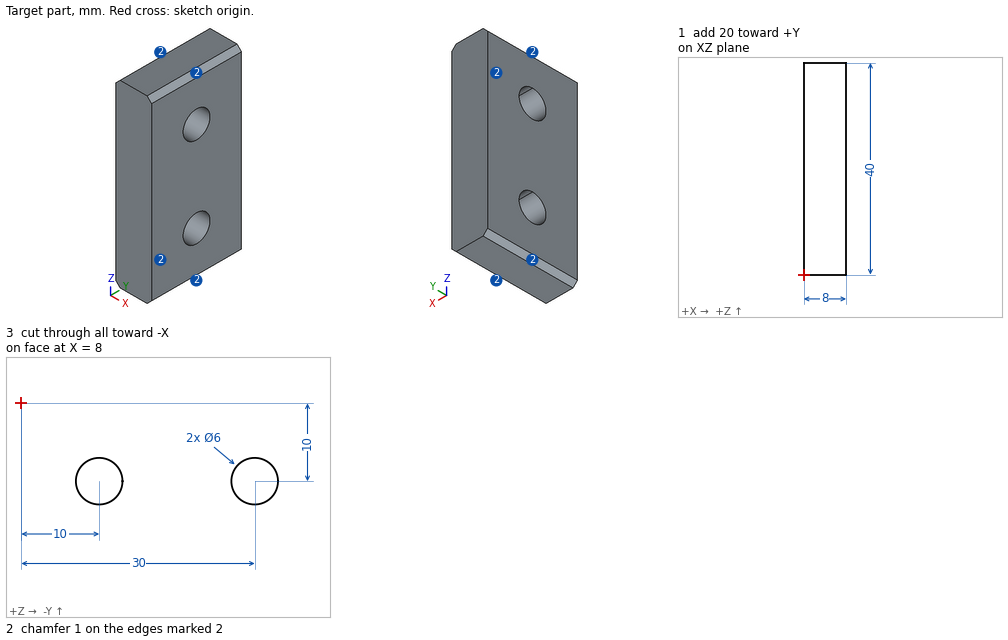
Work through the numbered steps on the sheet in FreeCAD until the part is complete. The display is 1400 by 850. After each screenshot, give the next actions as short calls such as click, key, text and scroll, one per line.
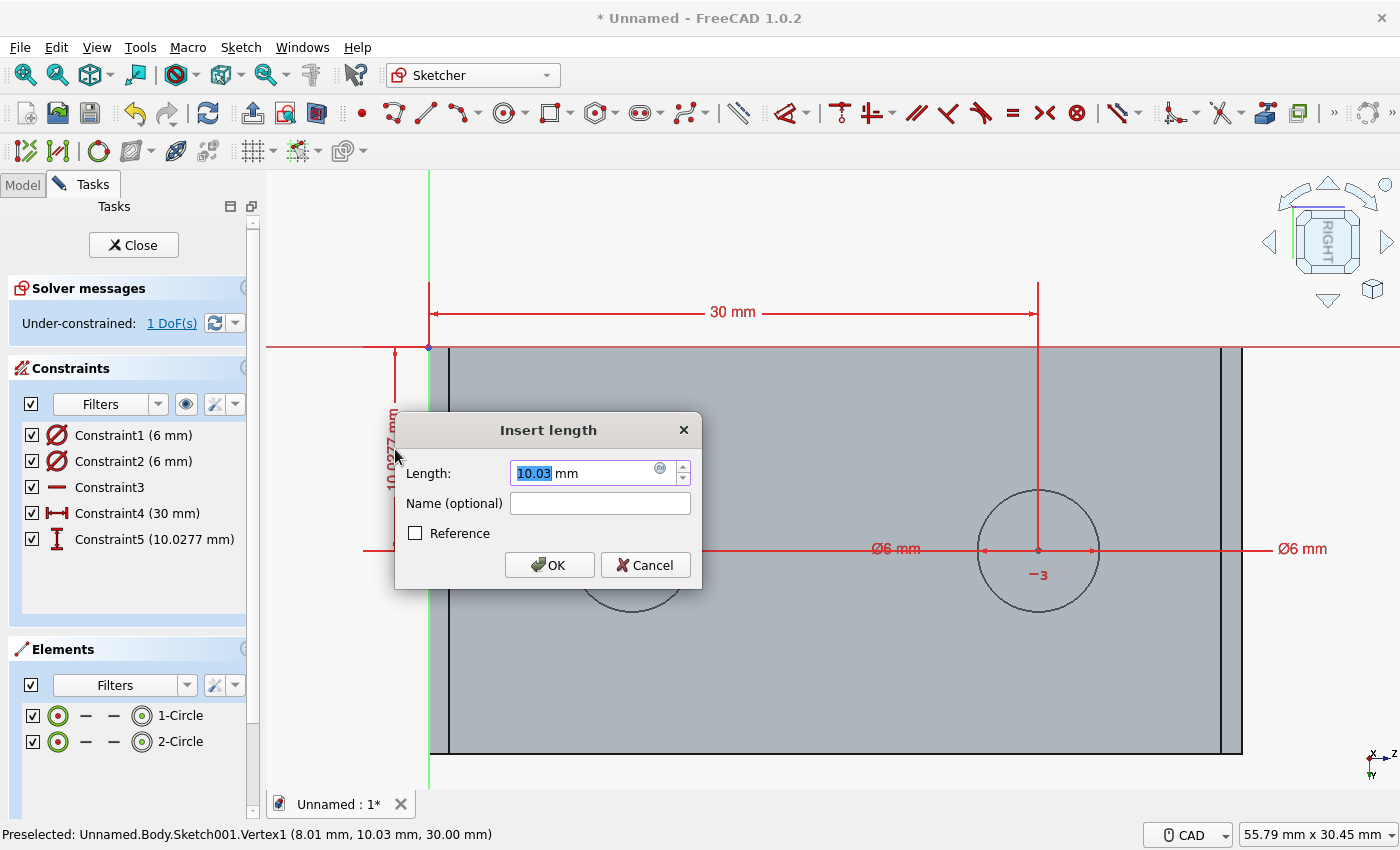
text(10)
key(Return)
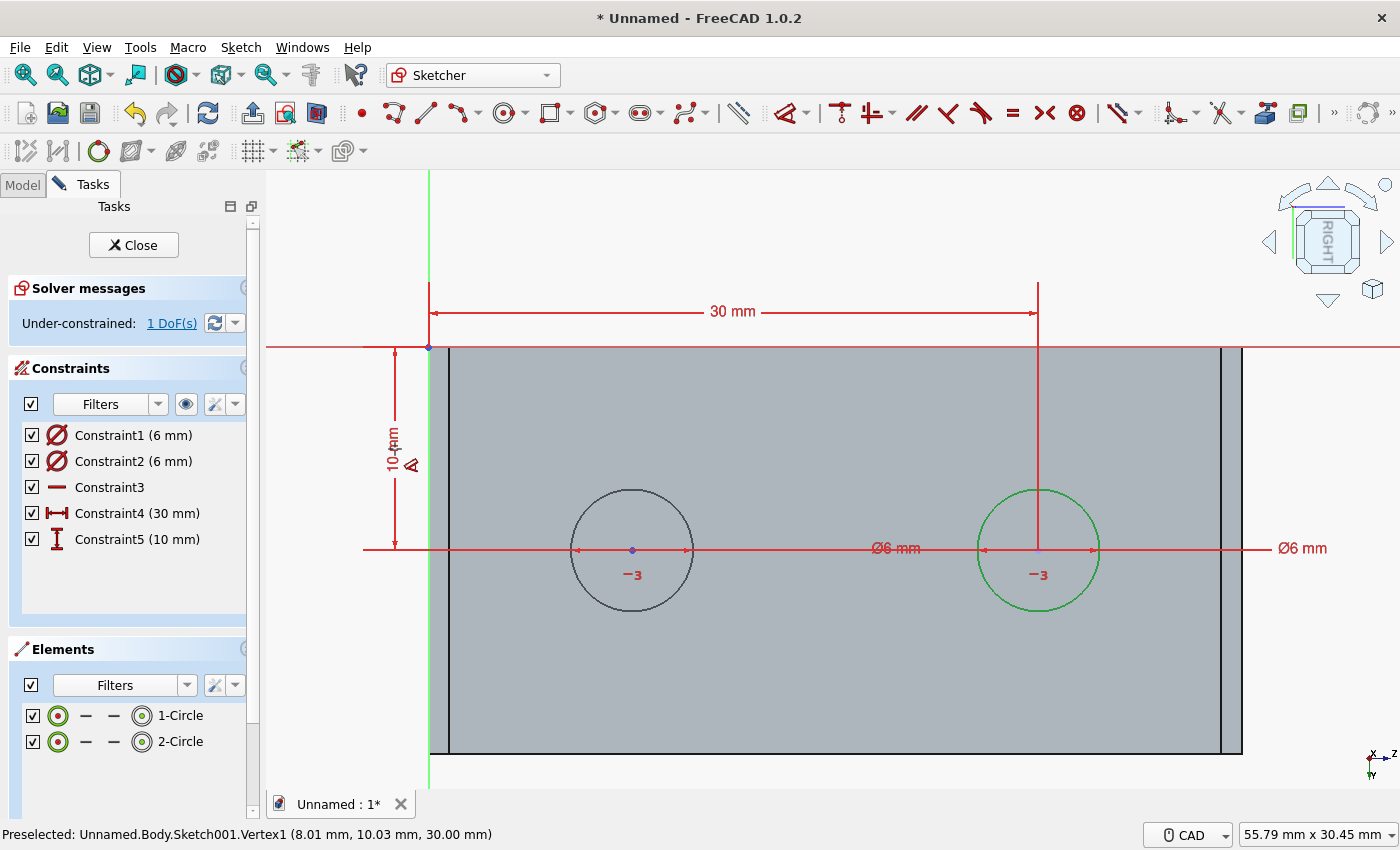
click(632, 550)
click(530, 313)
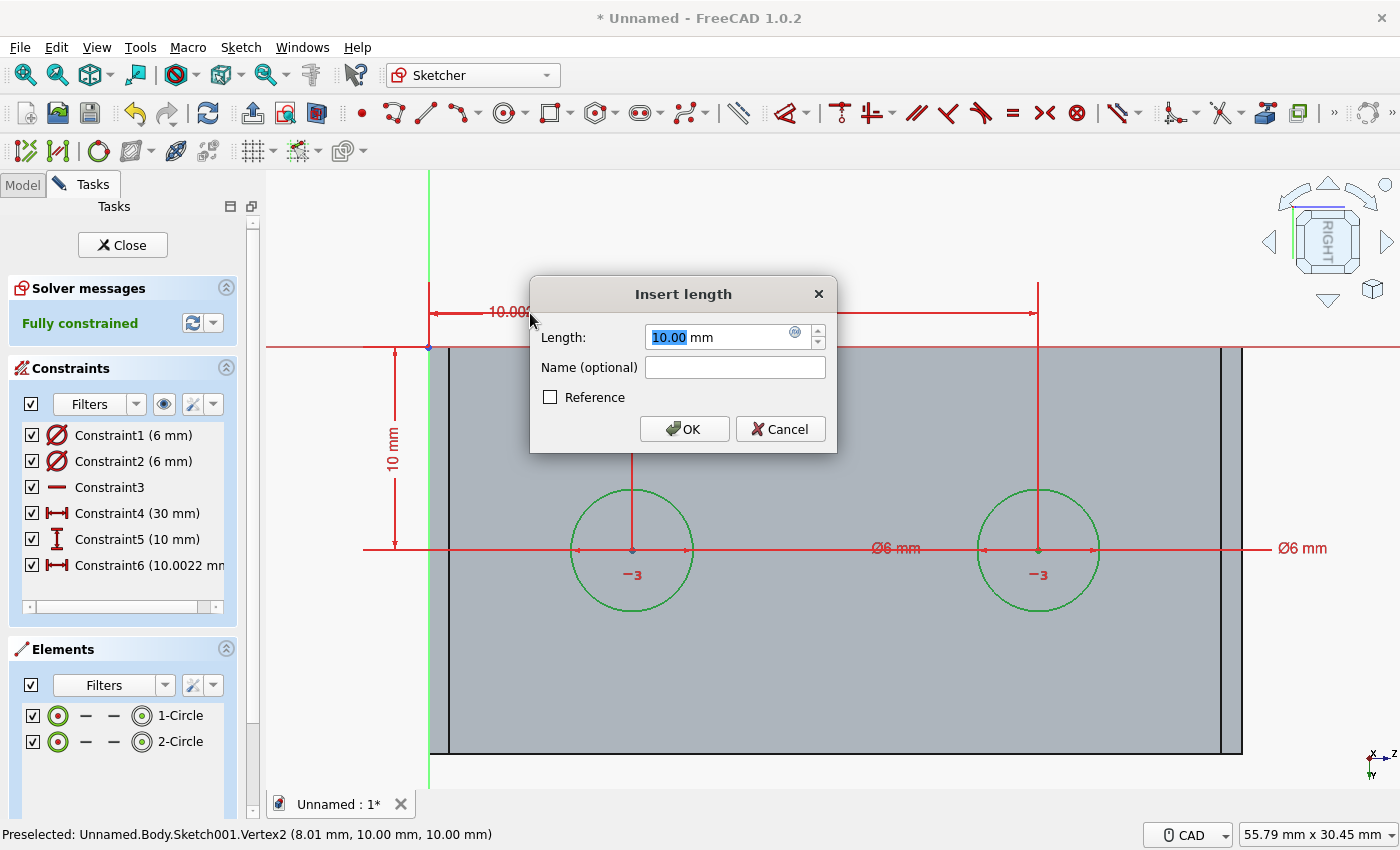
text(10)
key(Return)
key(Escape)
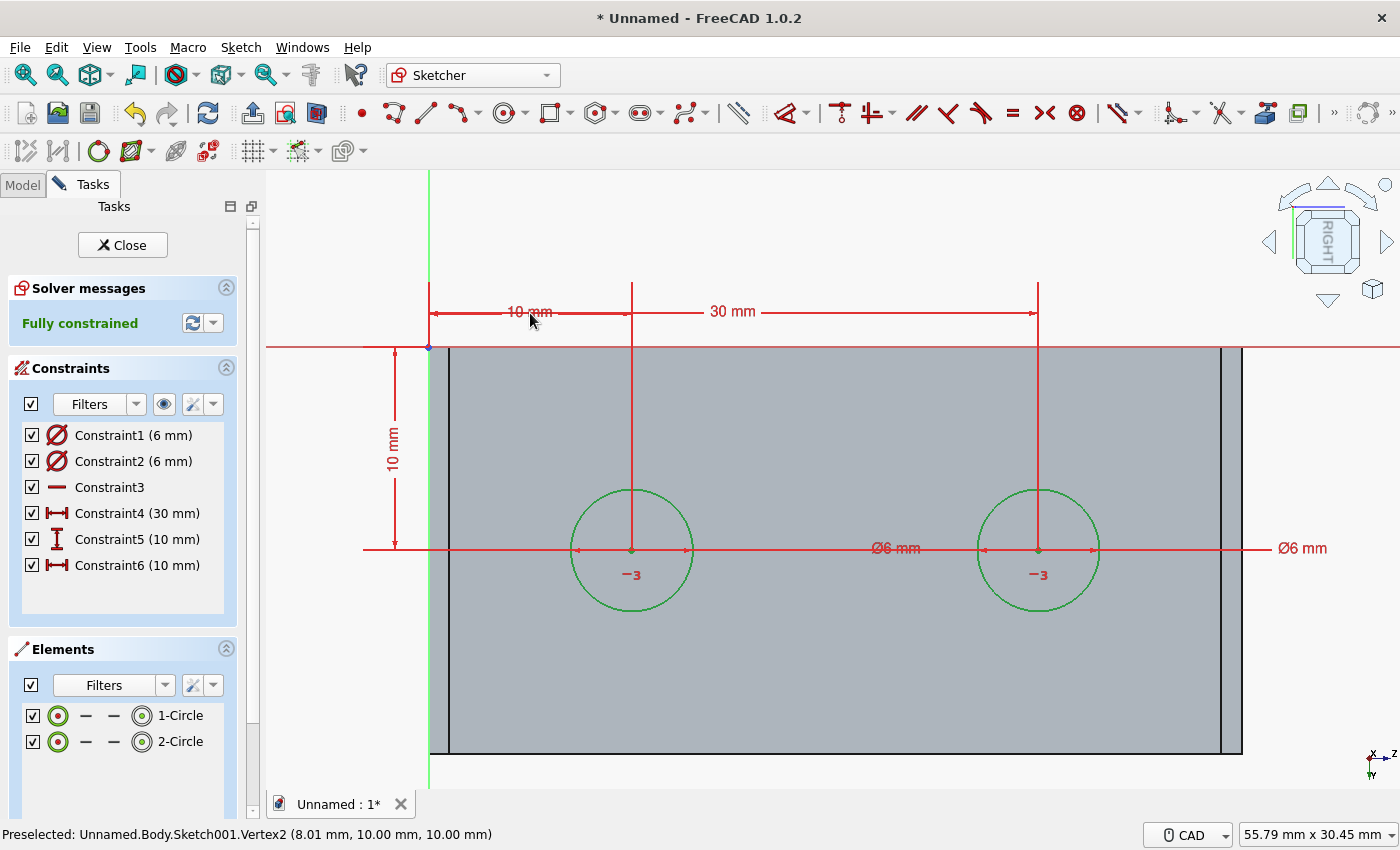
click(123, 245)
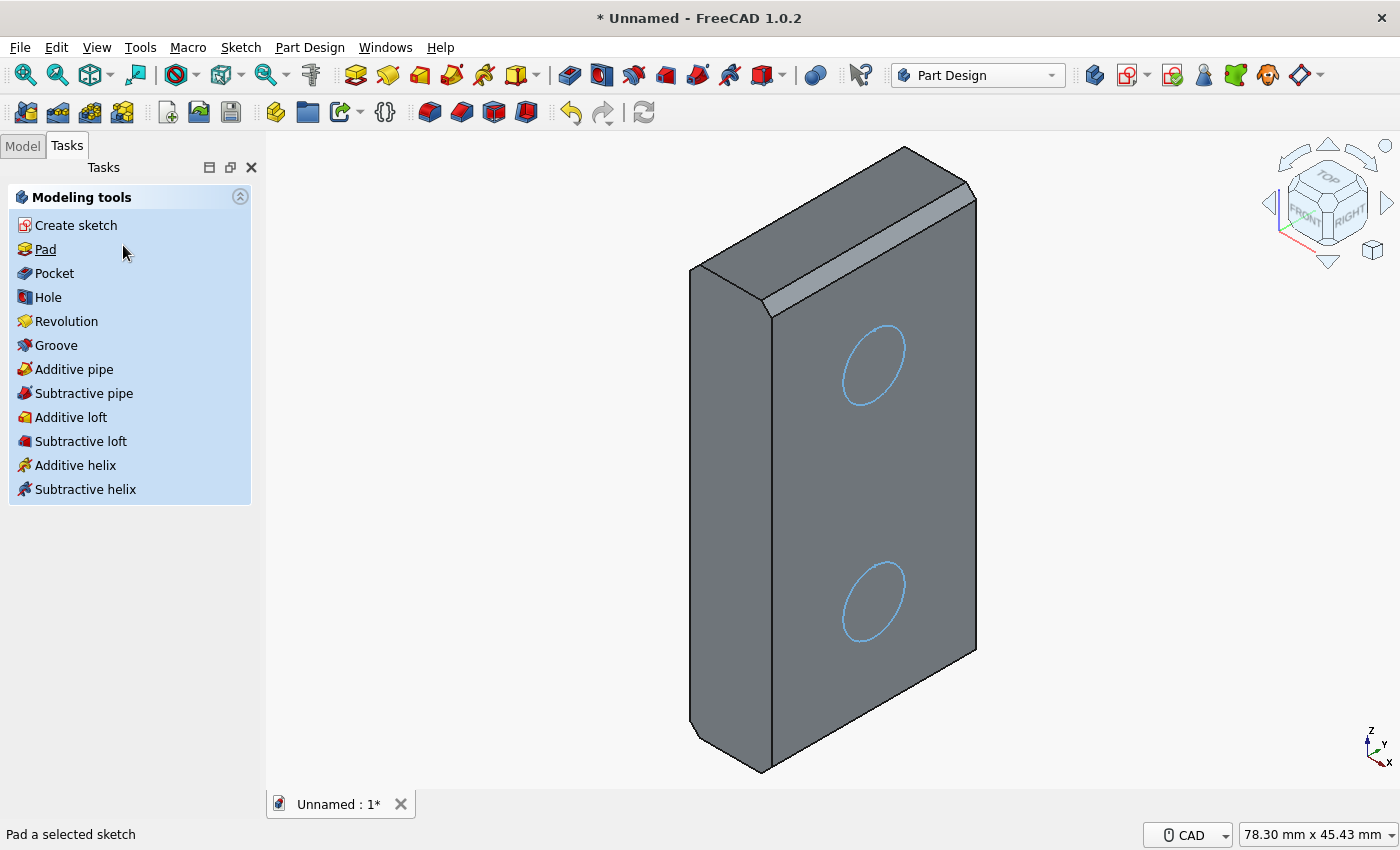
click(570, 76)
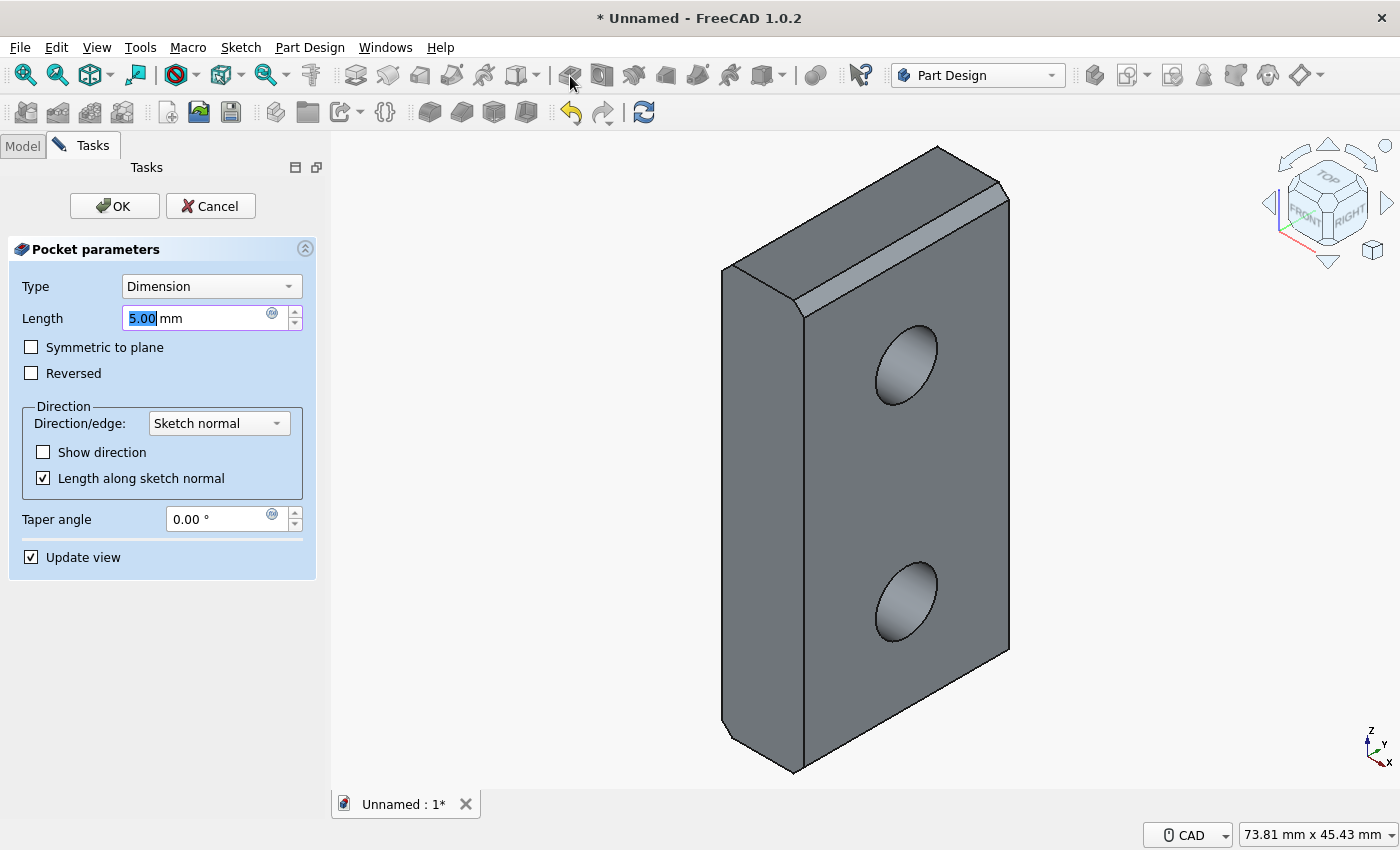
click(212, 286)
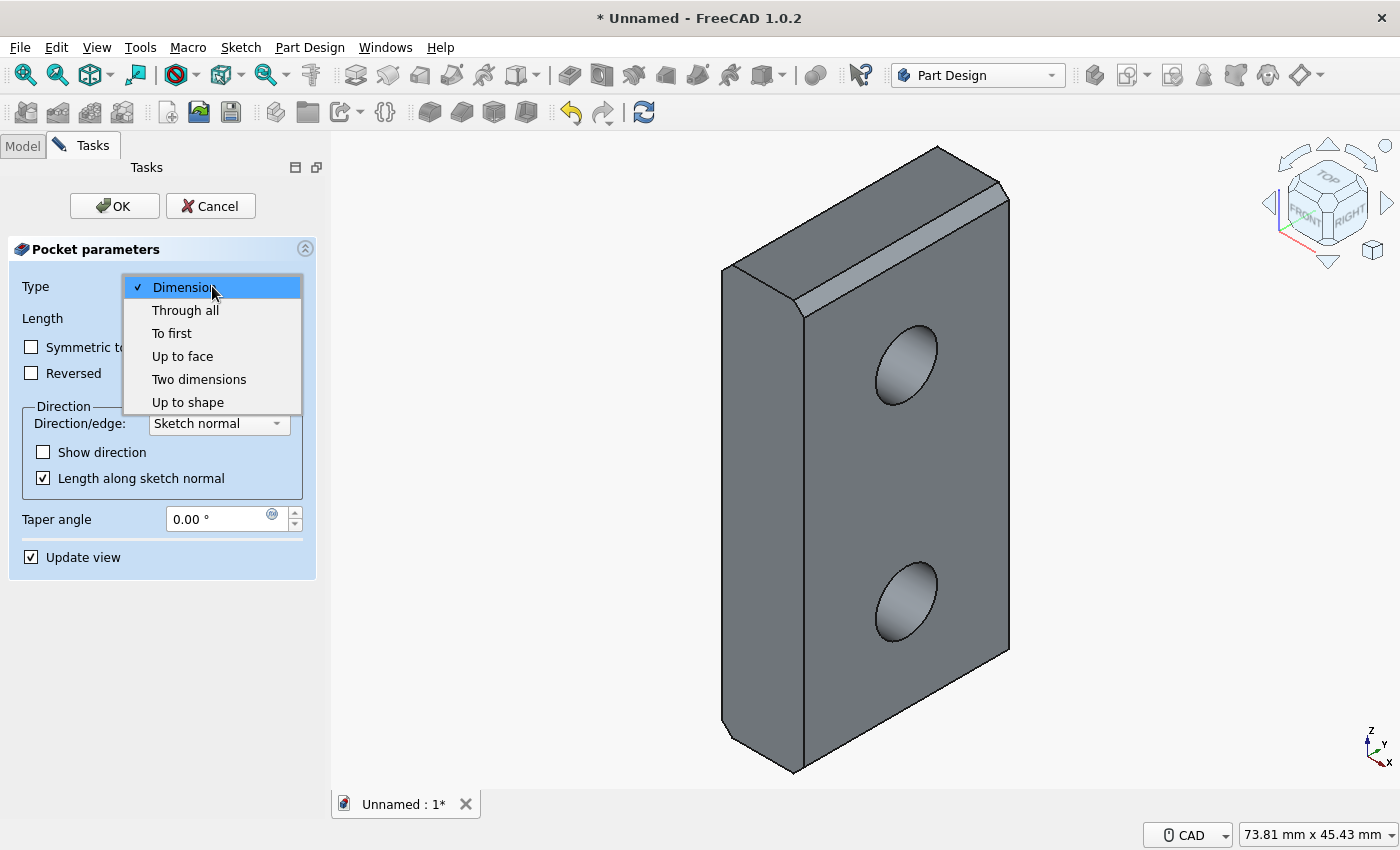
click(212, 310)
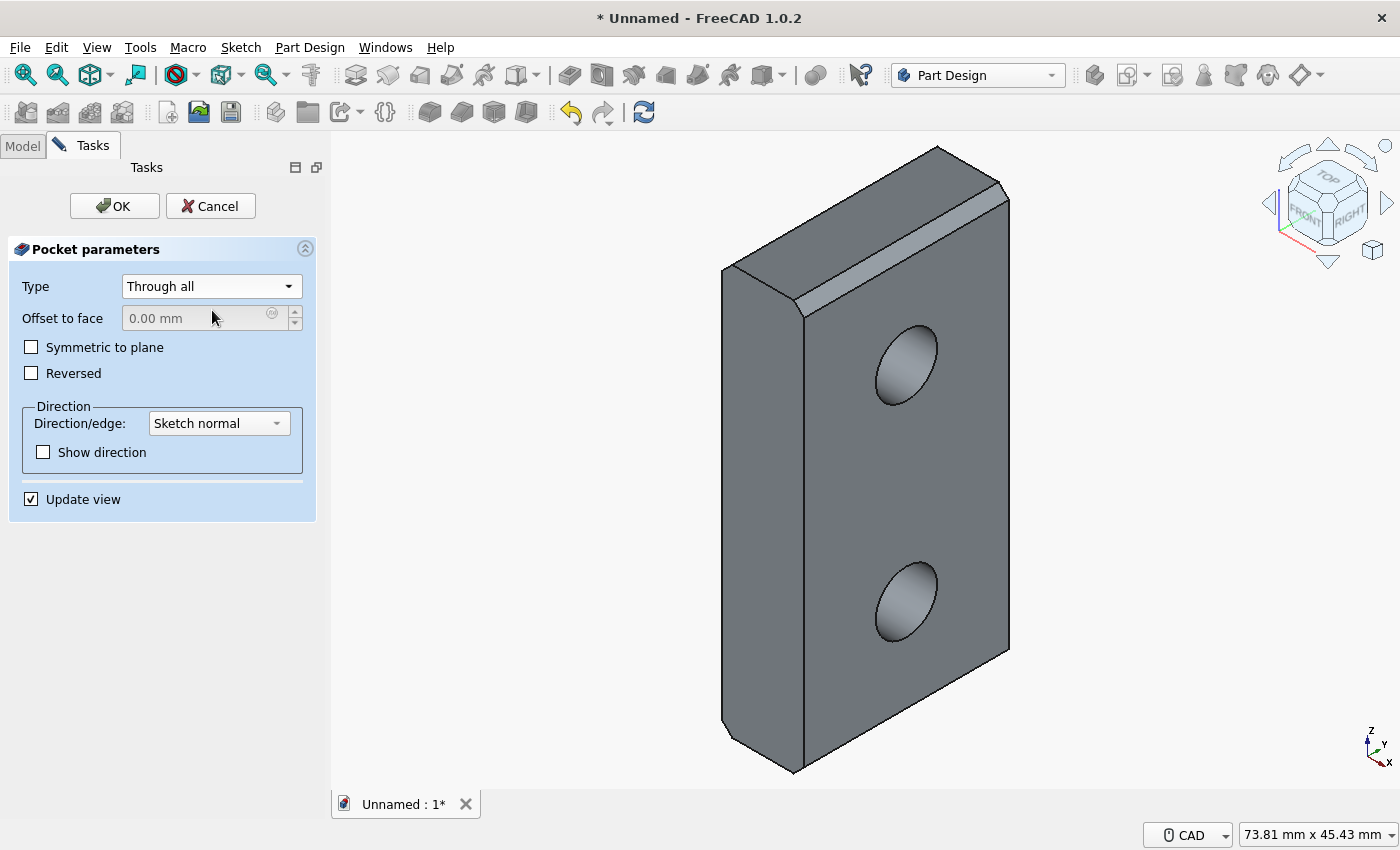
click(115, 206)